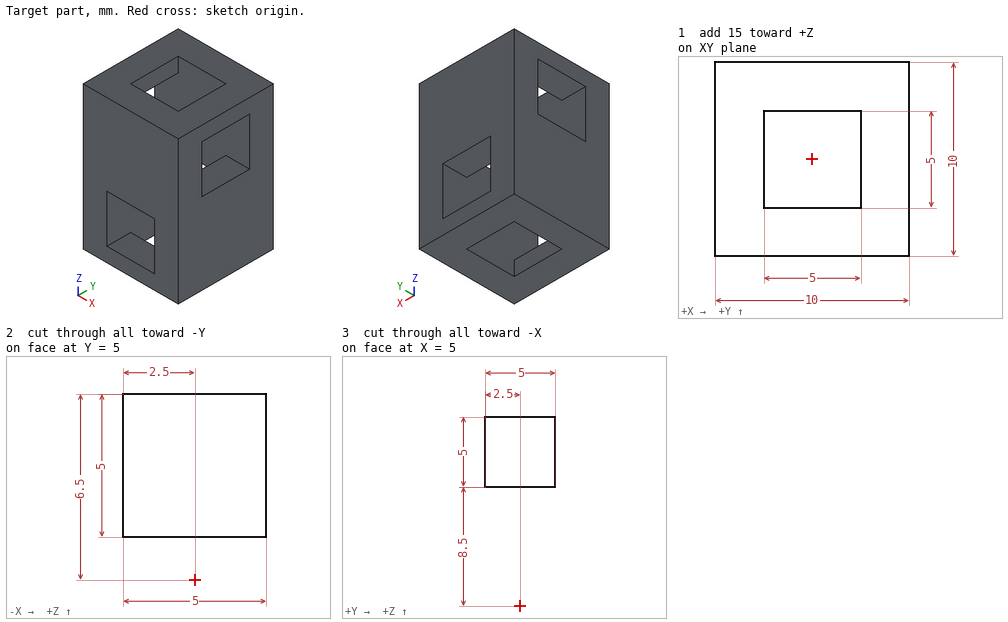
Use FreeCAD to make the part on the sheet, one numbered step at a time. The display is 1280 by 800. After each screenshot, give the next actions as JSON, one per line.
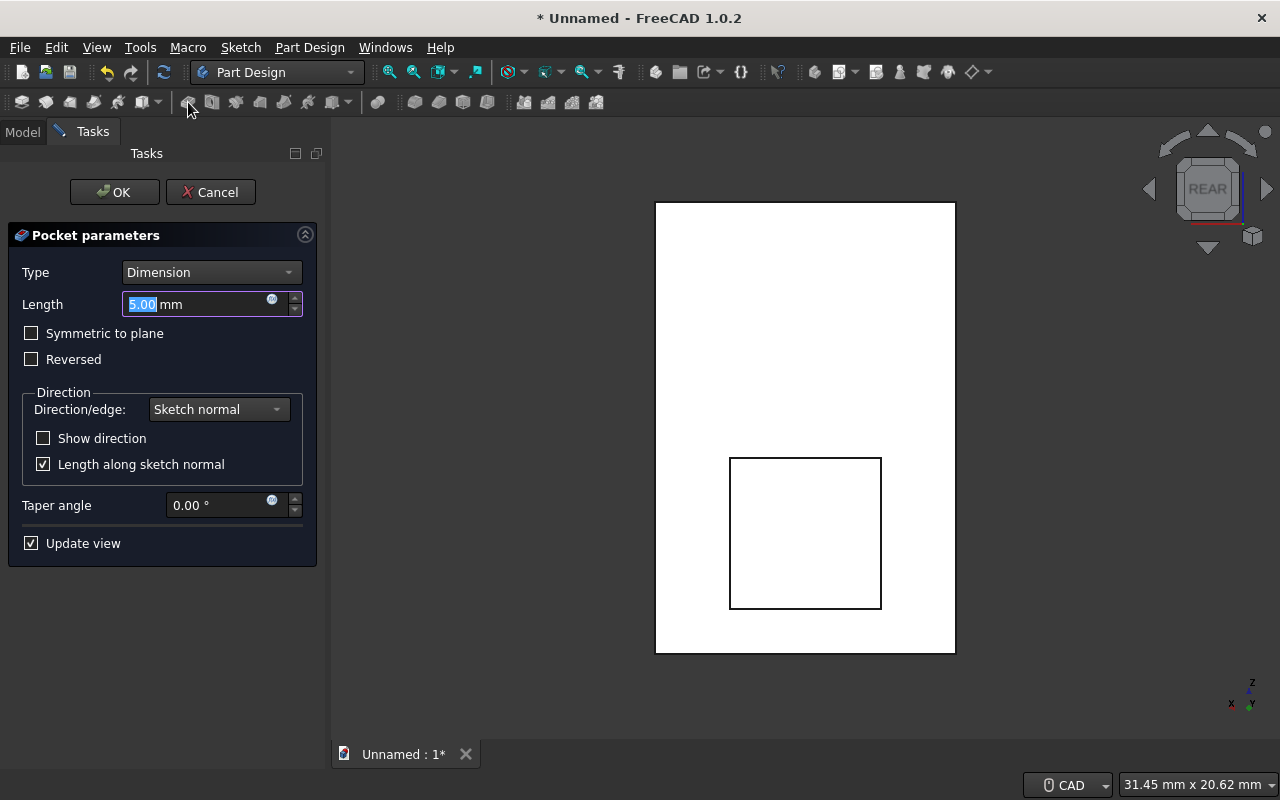
{"action": "left_click", "coordinate": [212, 272]}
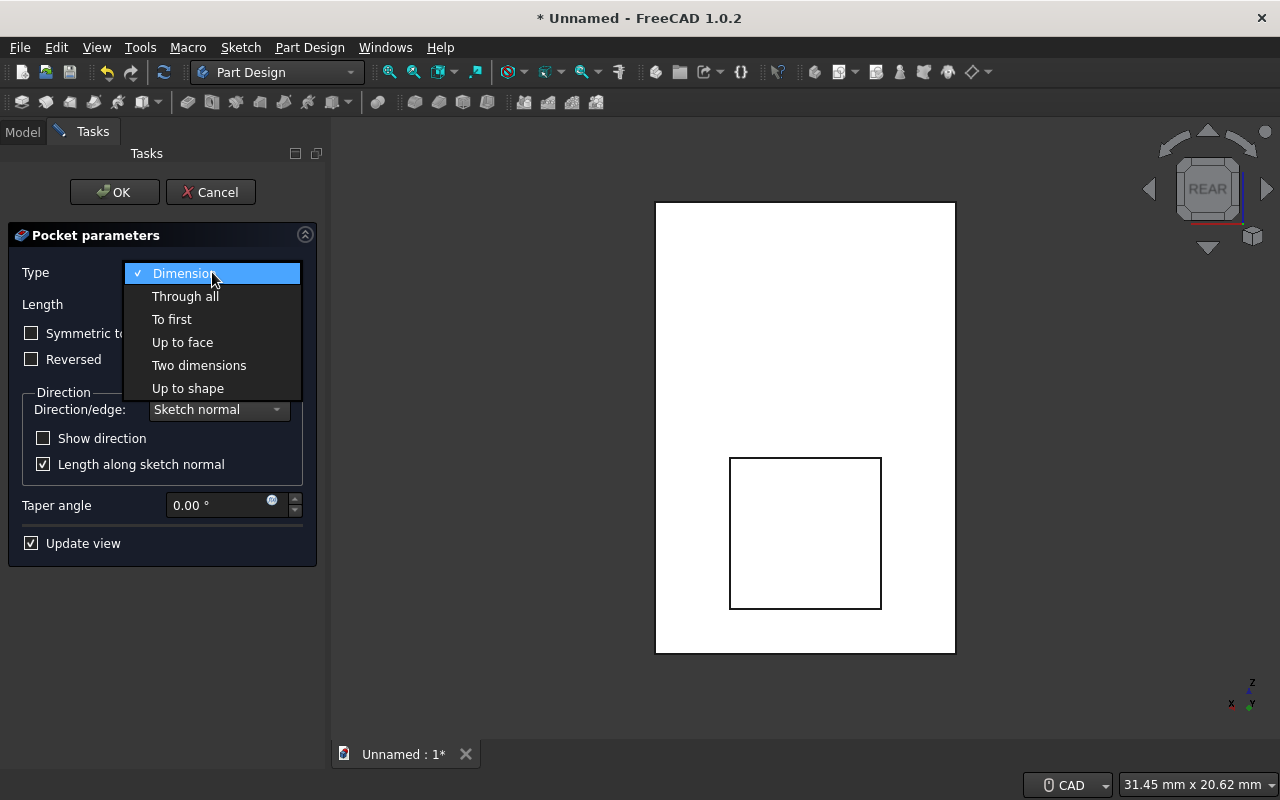
{"action": "left_click", "coordinate": [212, 296]}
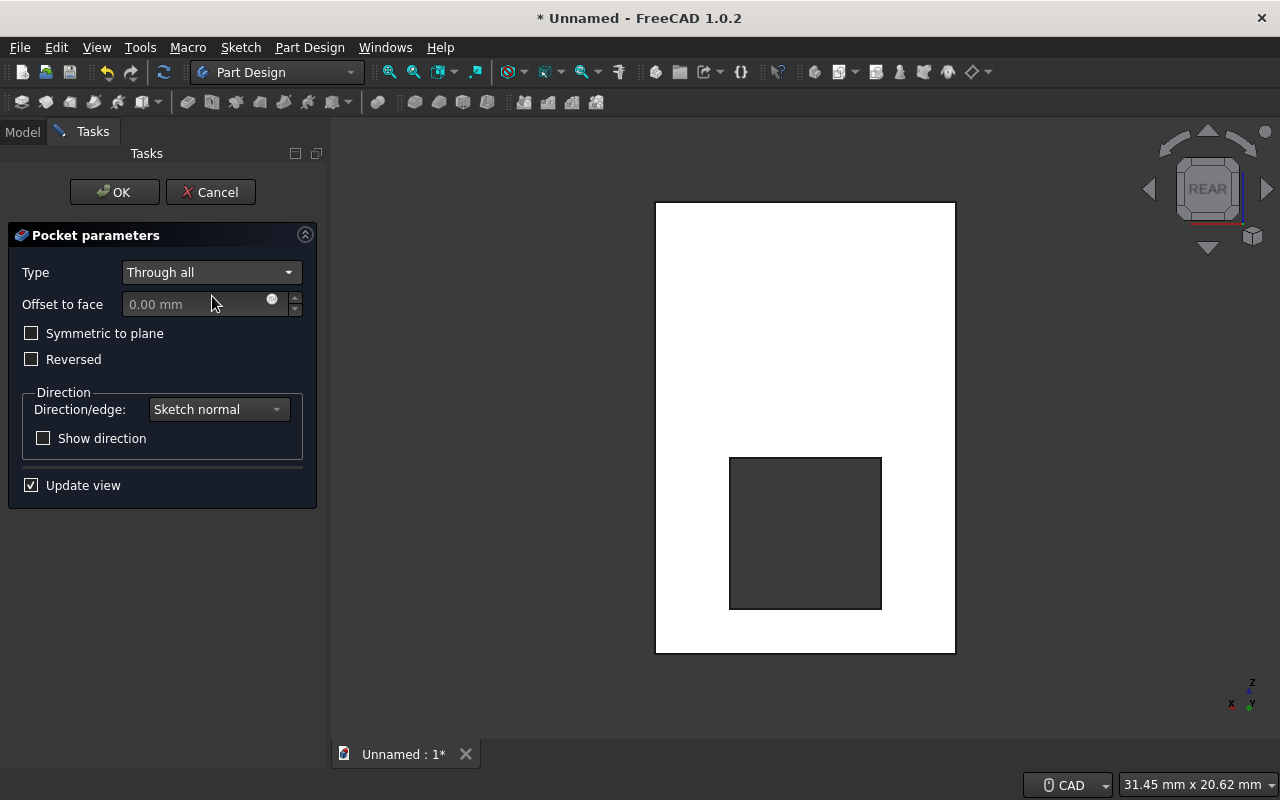
{"action": "left_click", "coordinate": [115, 192]}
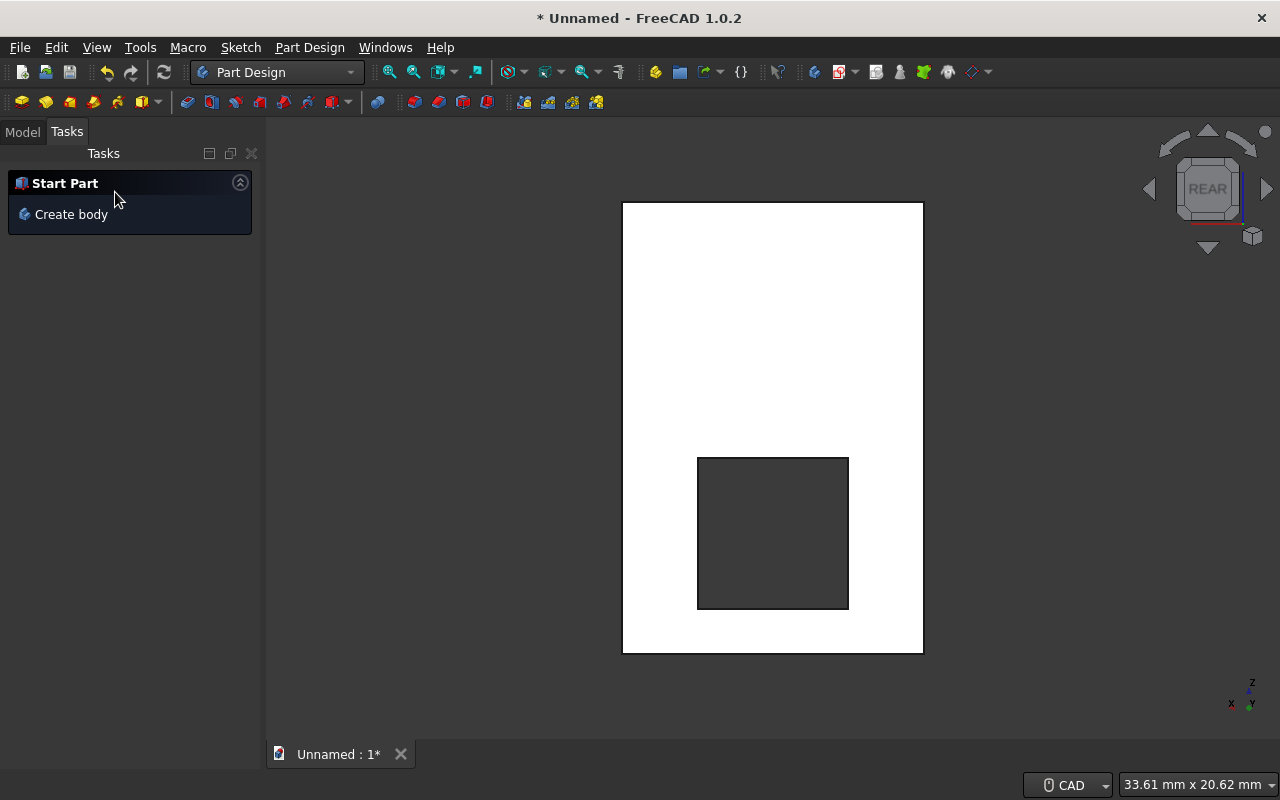
{"action": "key", "text": "0"}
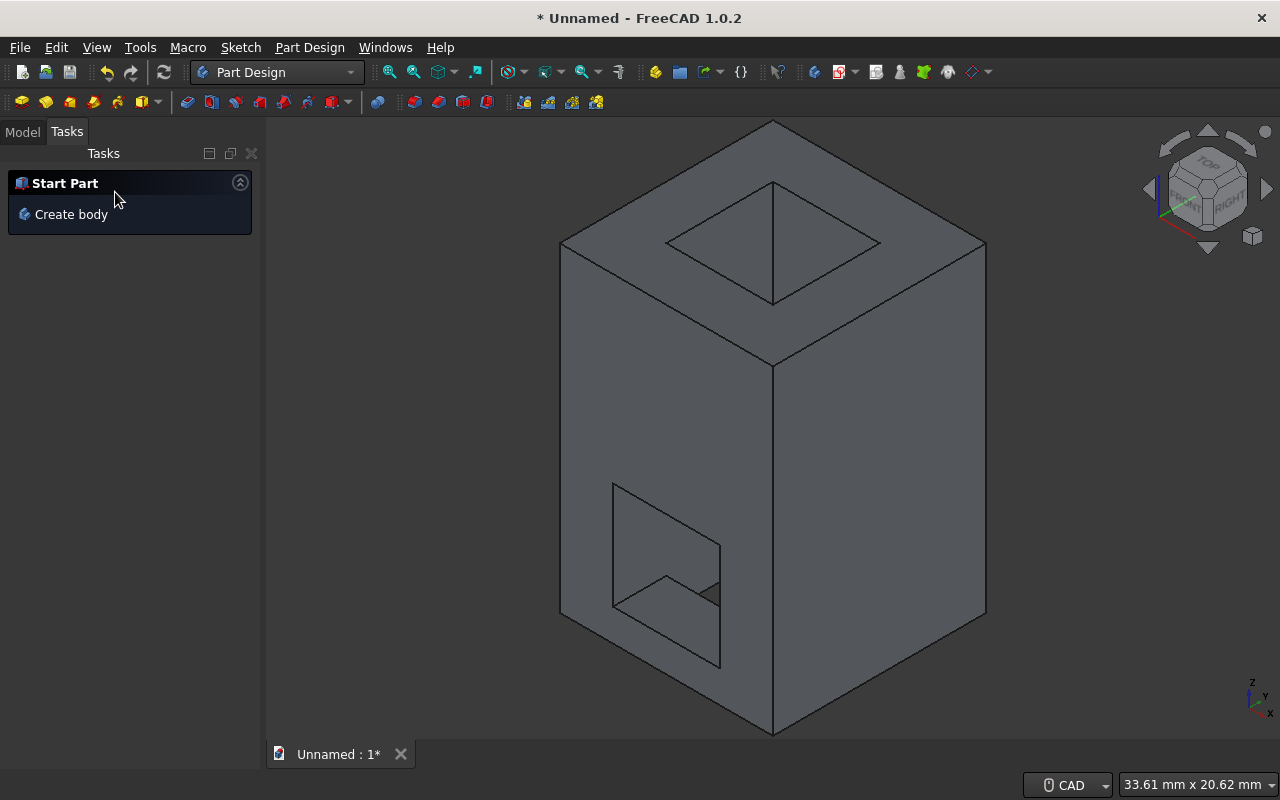
{"action": "left_click", "coordinate": [880, 436]}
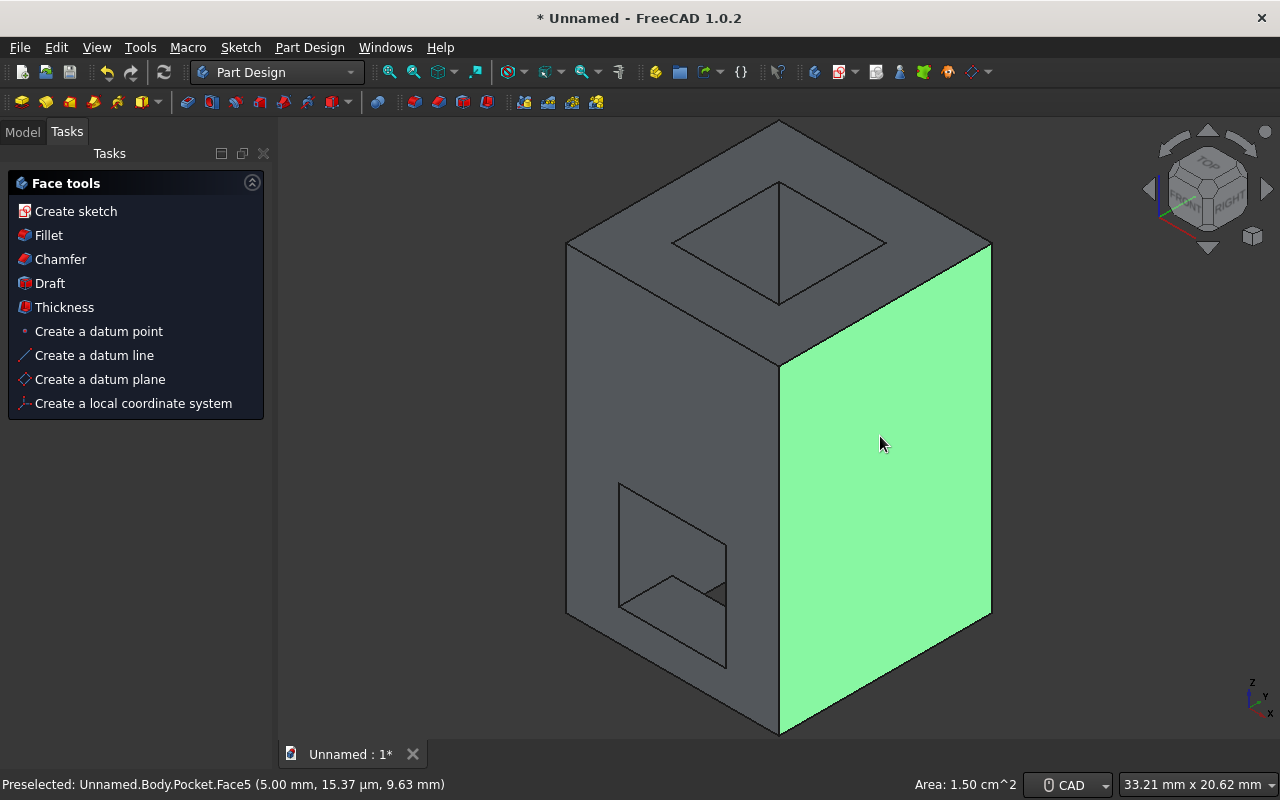
{"action": "left_click", "coordinate": [840, 72]}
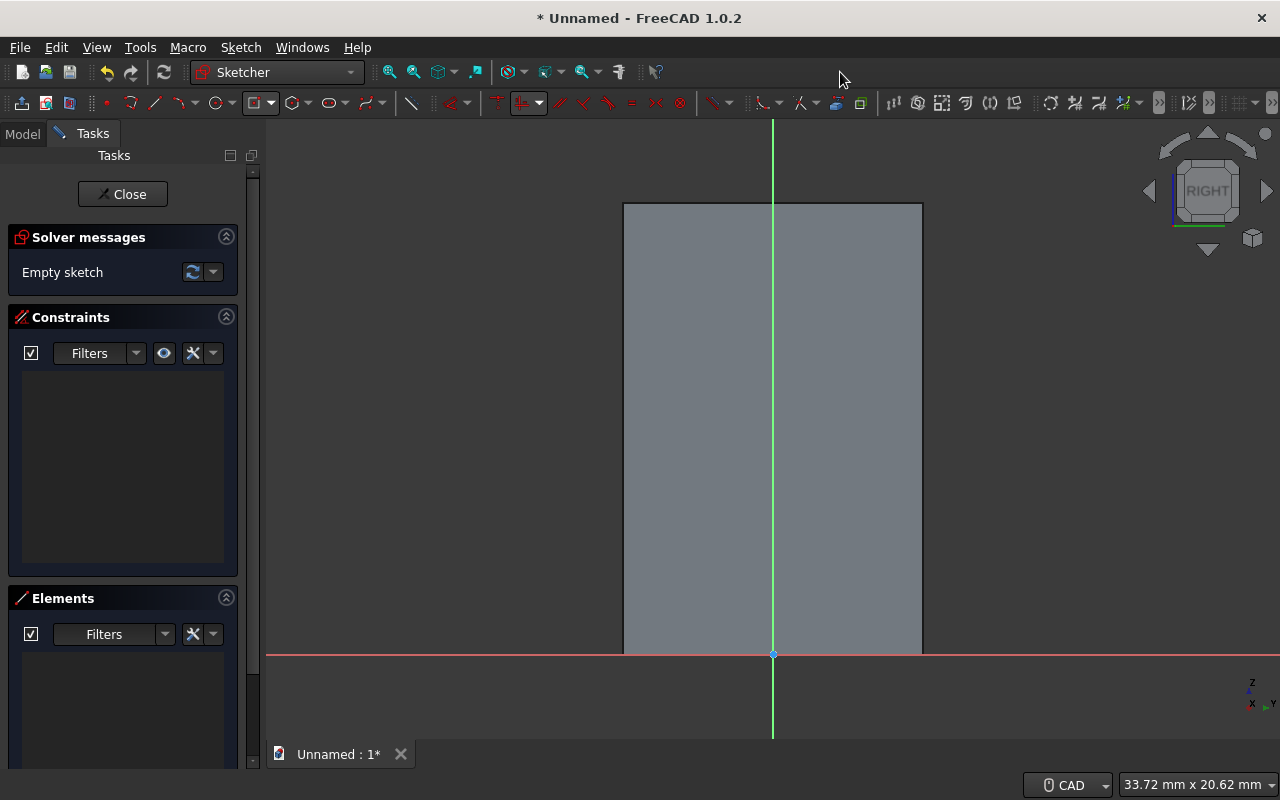
{"action": "scroll", "coordinate": [813, 262], "scroll_direction": "up", "scroll_amount": 5}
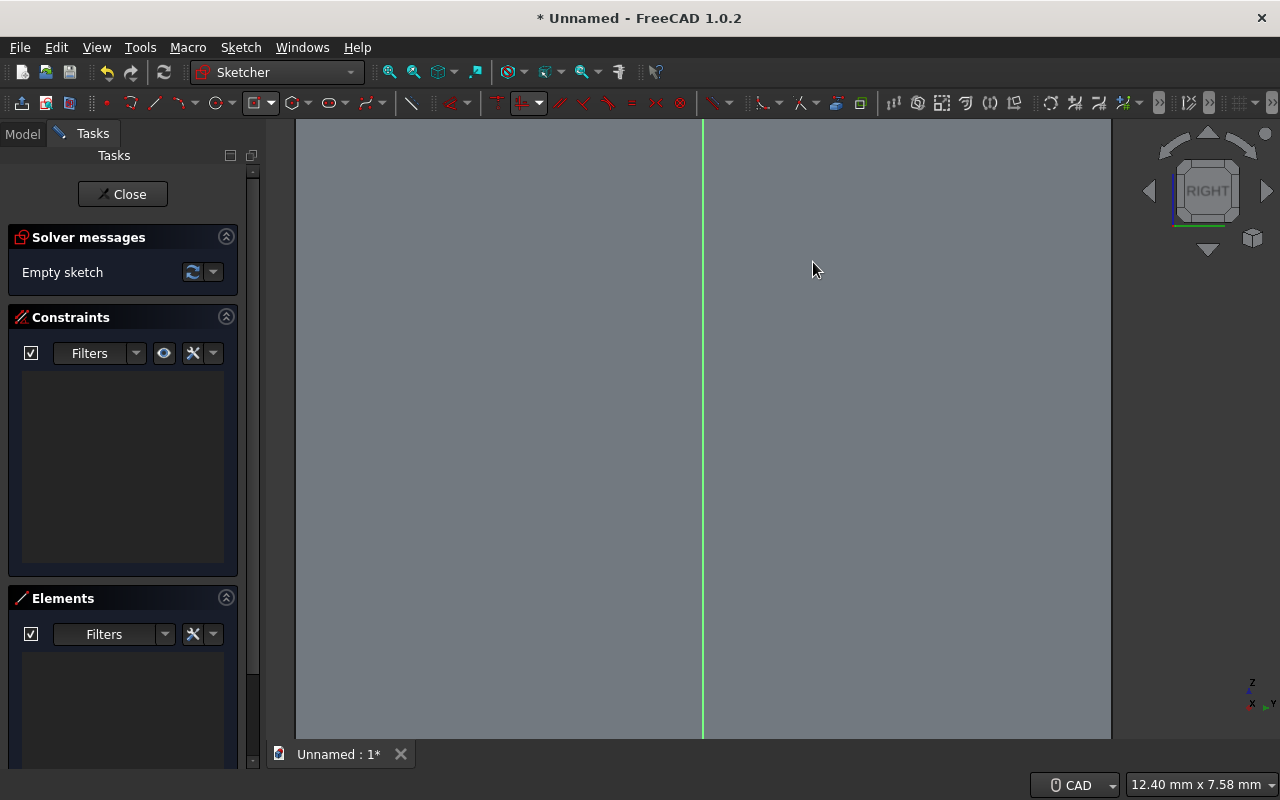
{"action": "left_click", "coordinate": [274, 104]}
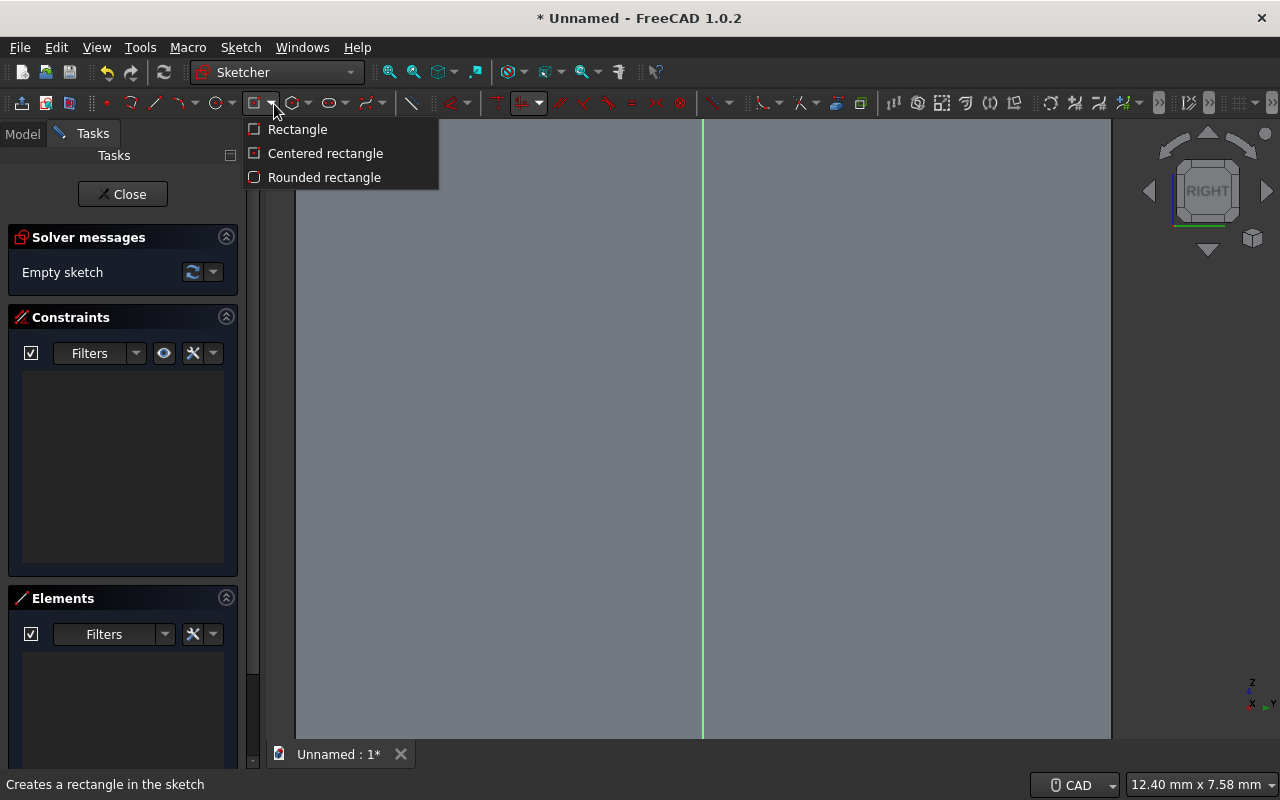
{"action": "left_click", "coordinate": [340, 129]}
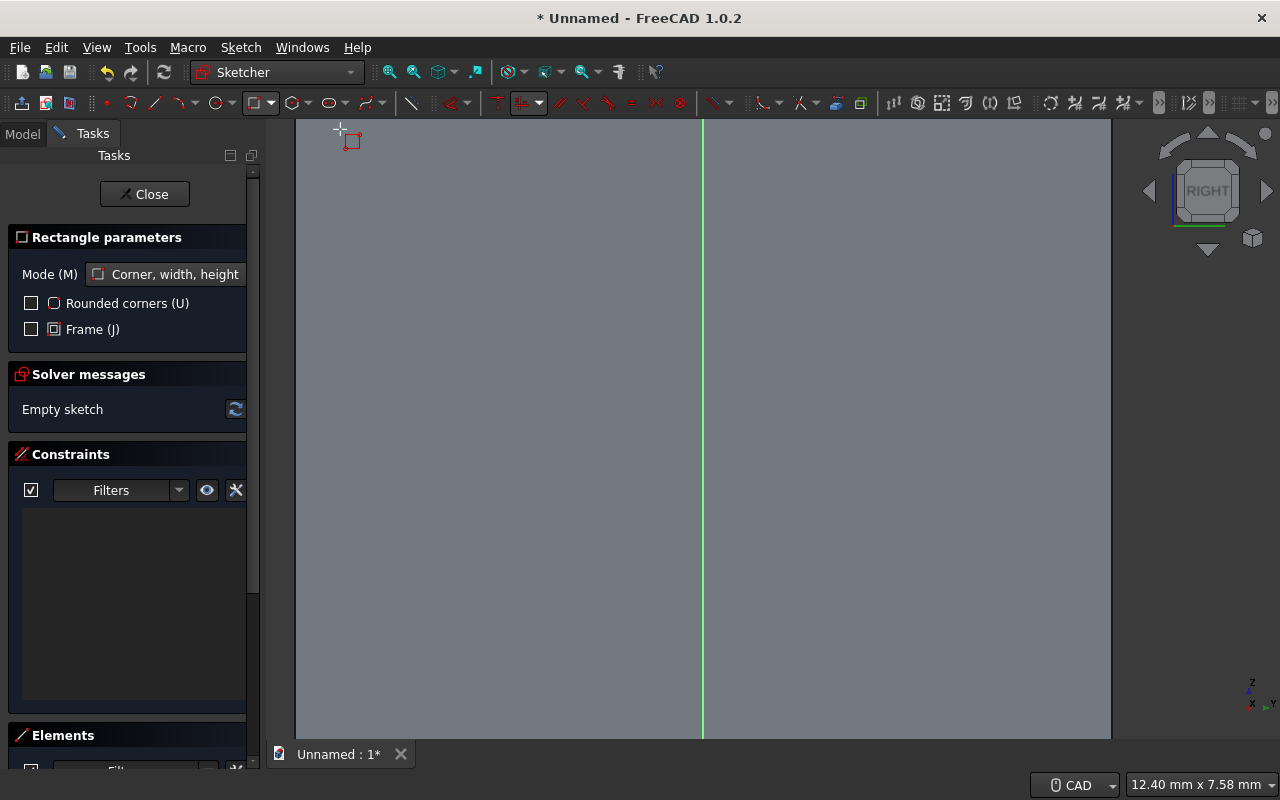
{"action": "left_click", "coordinate": [499, 225]}
{"action": "left_click", "coordinate": [908, 634]}
{"action": "key", "text": "Escape"}